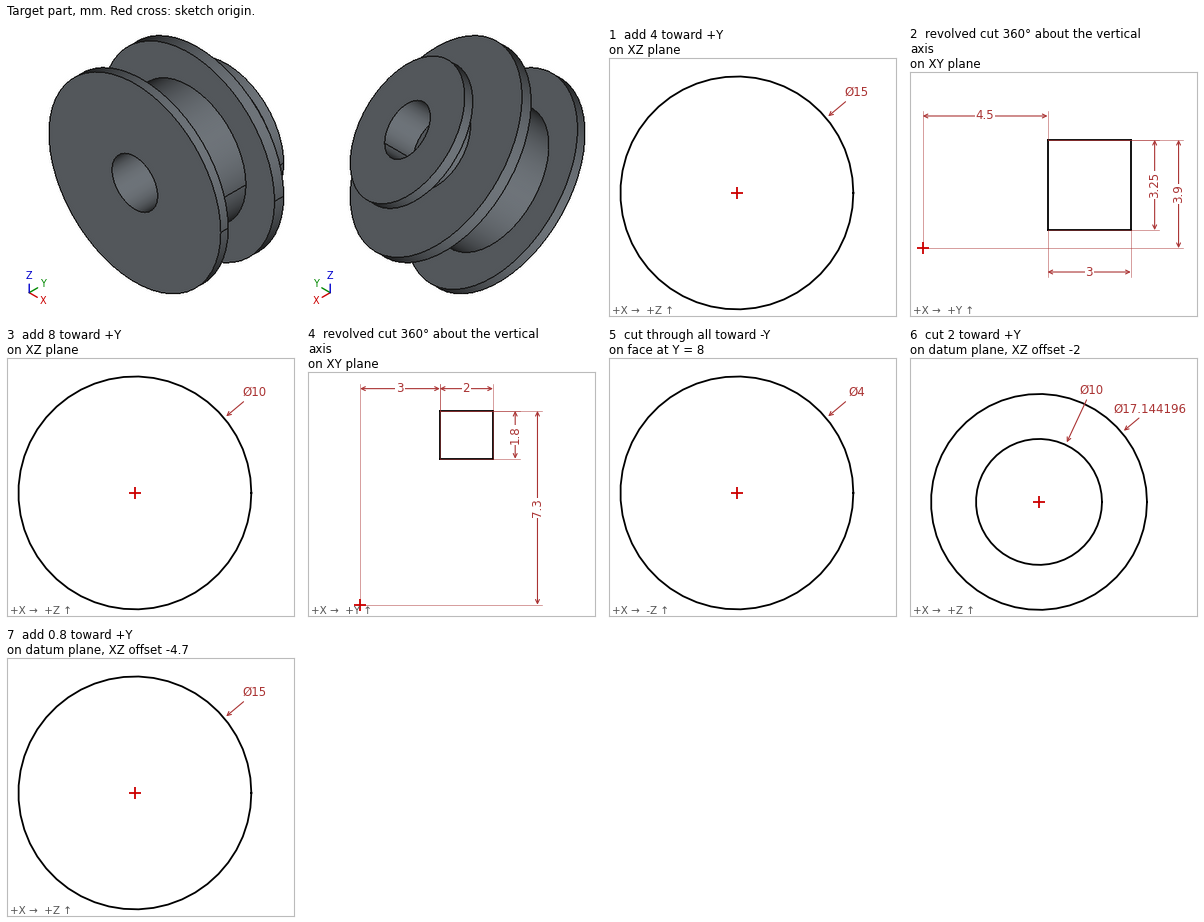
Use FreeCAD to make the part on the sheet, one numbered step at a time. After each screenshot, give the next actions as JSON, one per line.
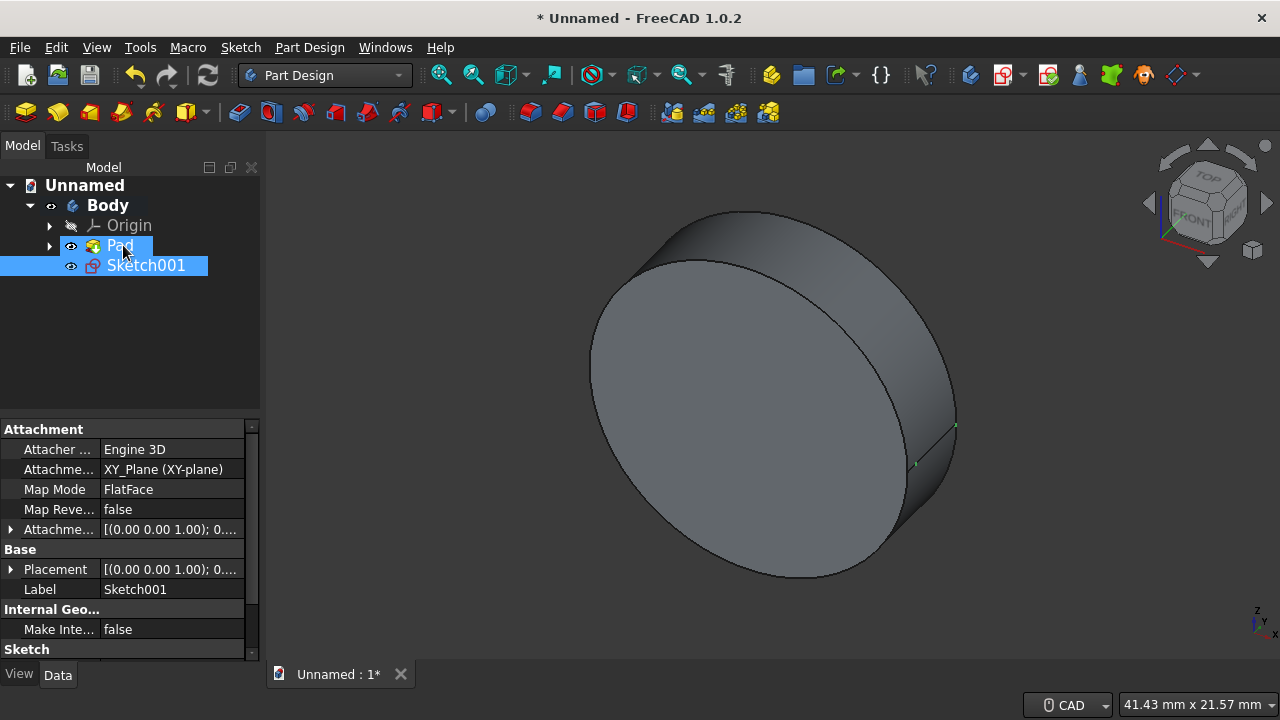
{"action": "left_click", "coordinate": [304, 112]}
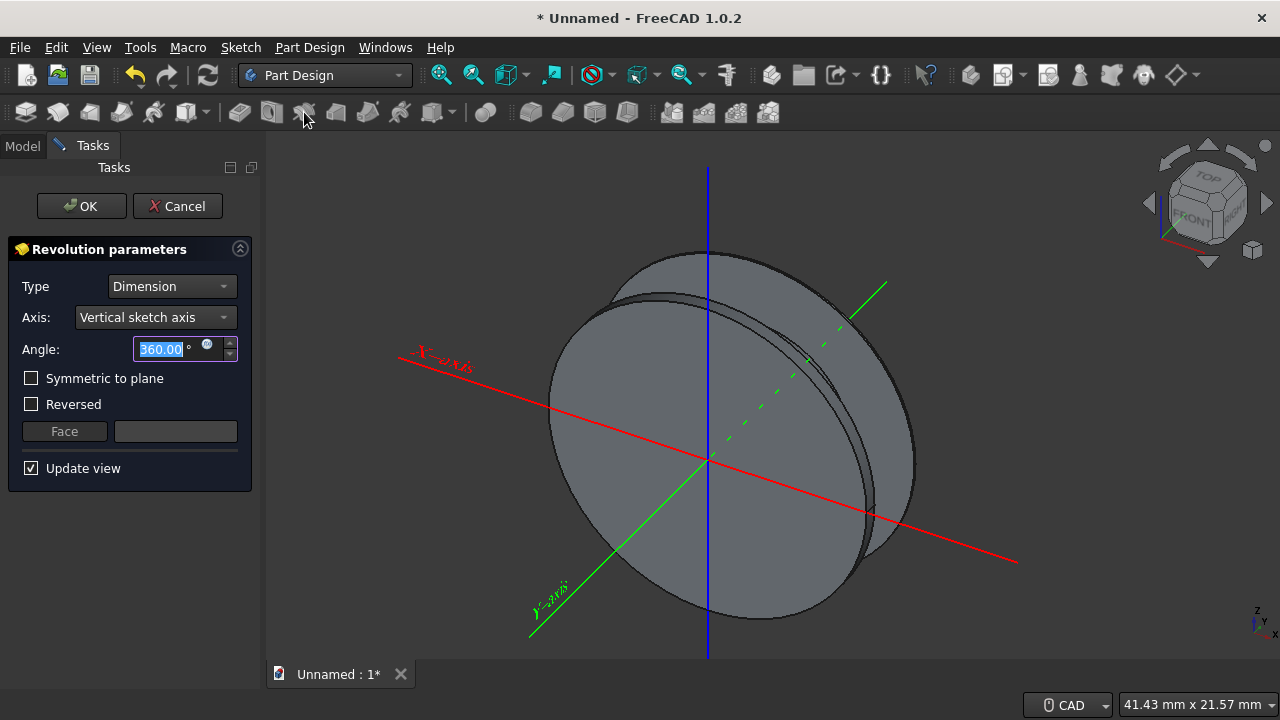
{"action": "left_click", "coordinate": [82, 206]}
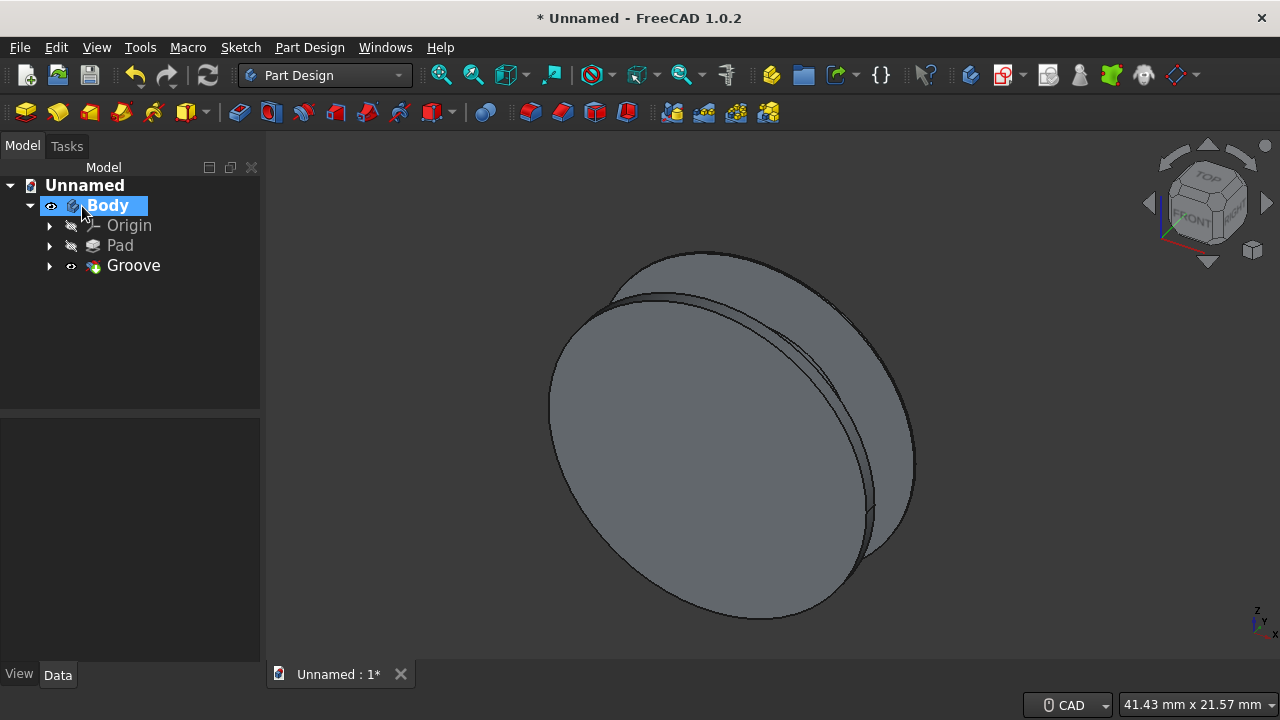
{"action": "left_click", "coordinate": [442, 76]}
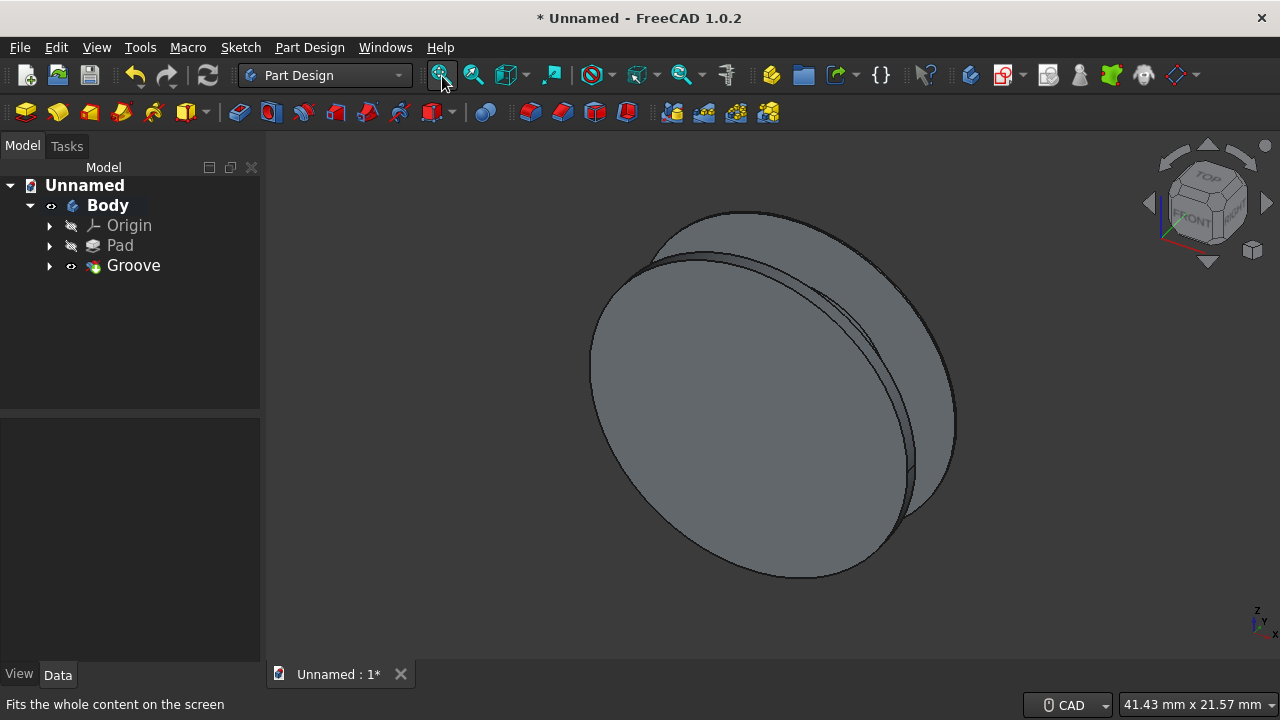
{"action": "left_click", "coordinate": [1004, 76]}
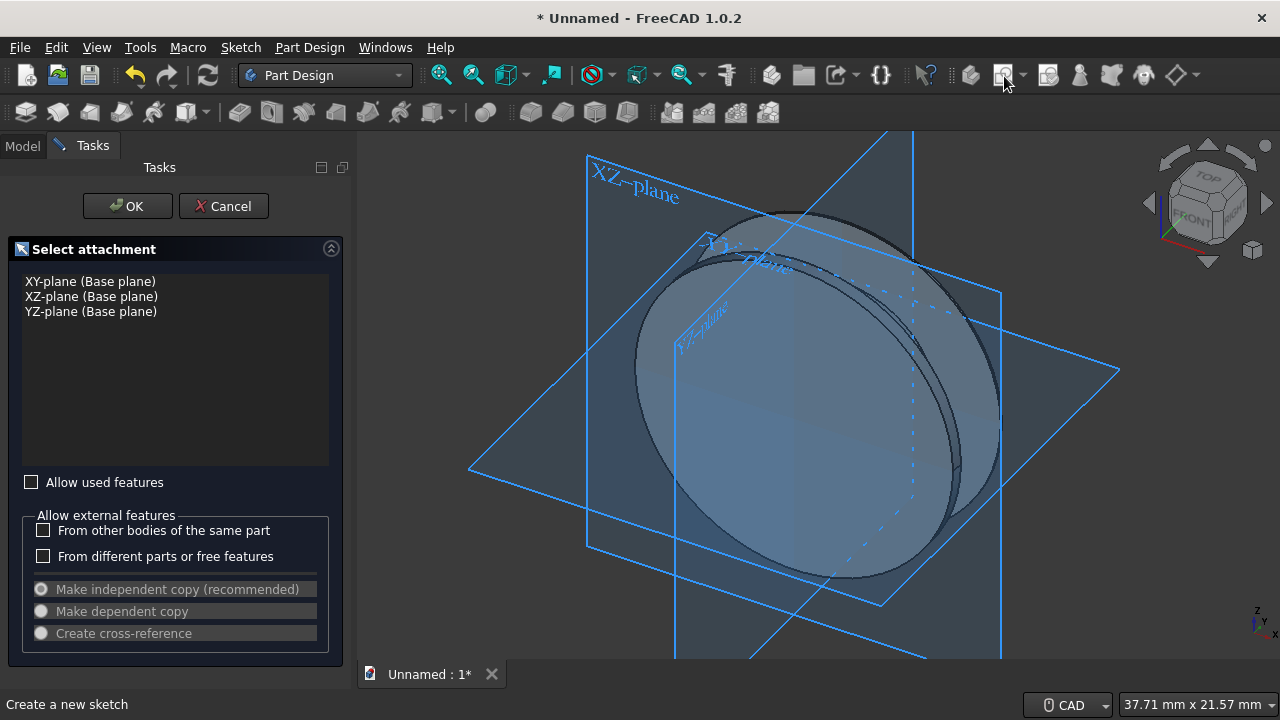
{"action": "left_click", "coordinate": [82, 296]}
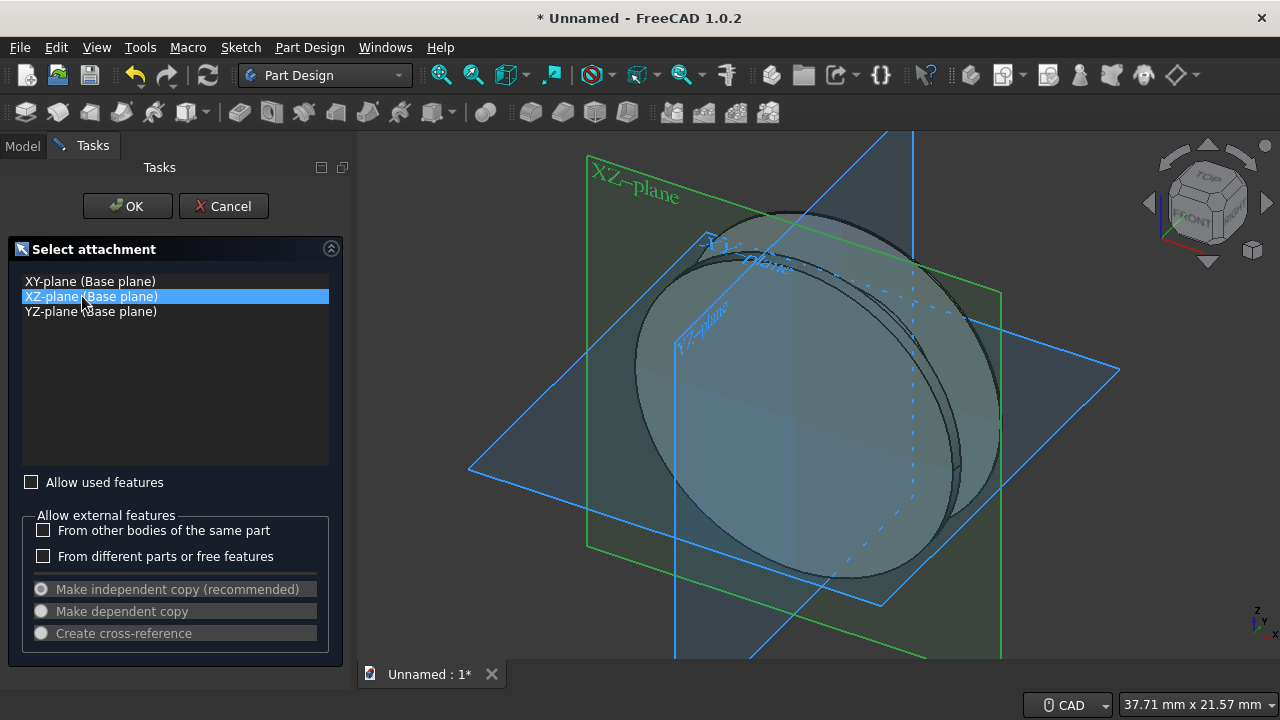
{"action": "left_click", "coordinate": [128, 206]}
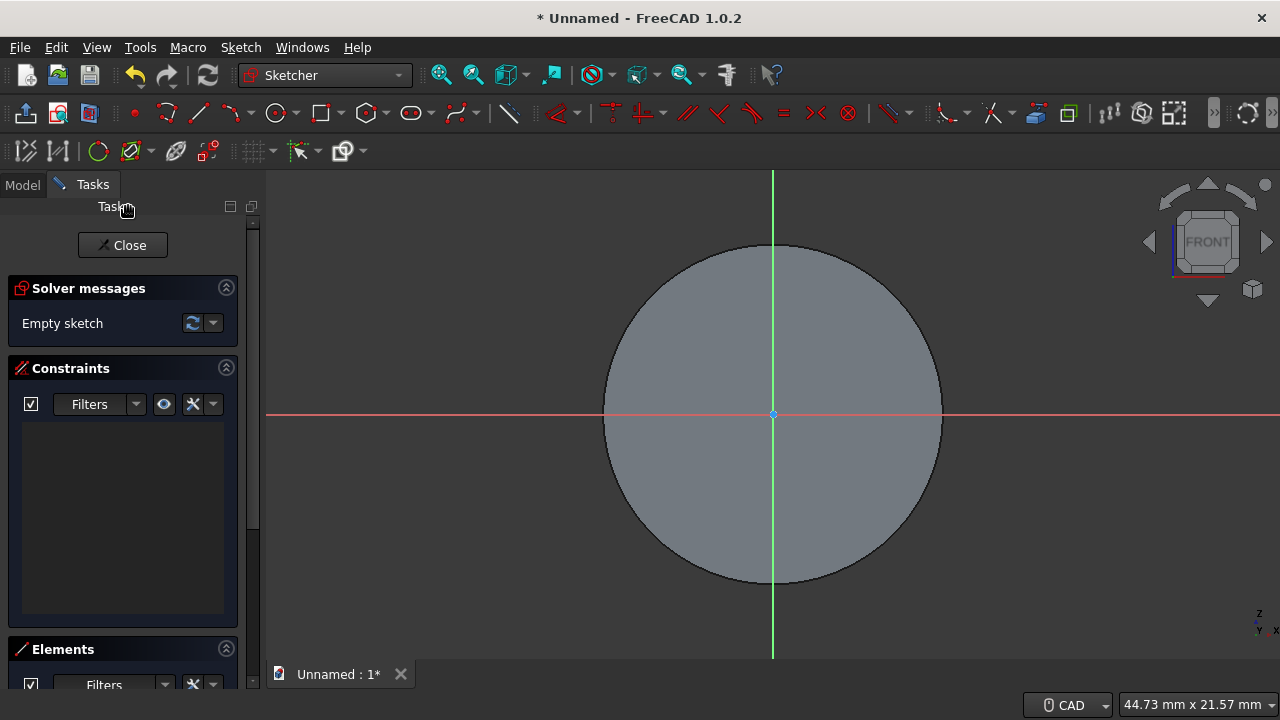
{"action": "left_click", "coordinate": [276, 114]}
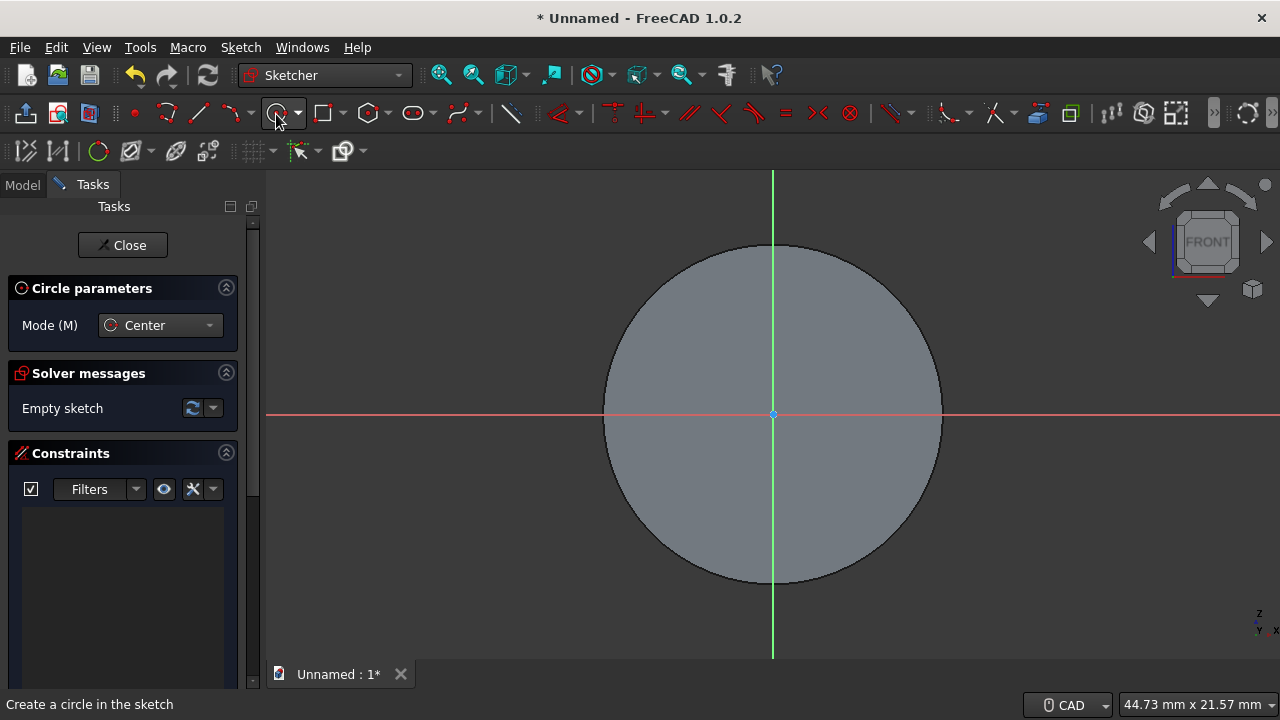
{"action": "left_click", "coordinate": [773, 414]}
{"action": "left_click", "coordinate": [853, 334]}
{"action": "key", "text": "Escape"}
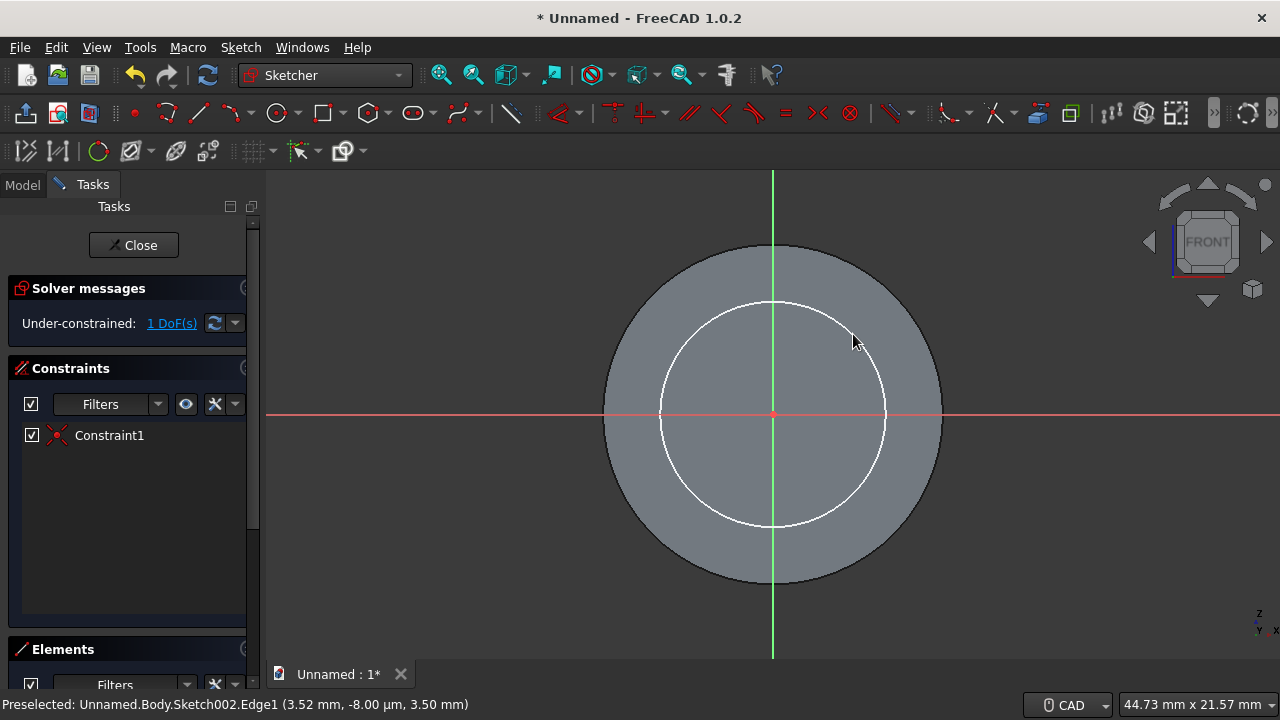
{"action": "left_click", "coordinate": [558, 114]}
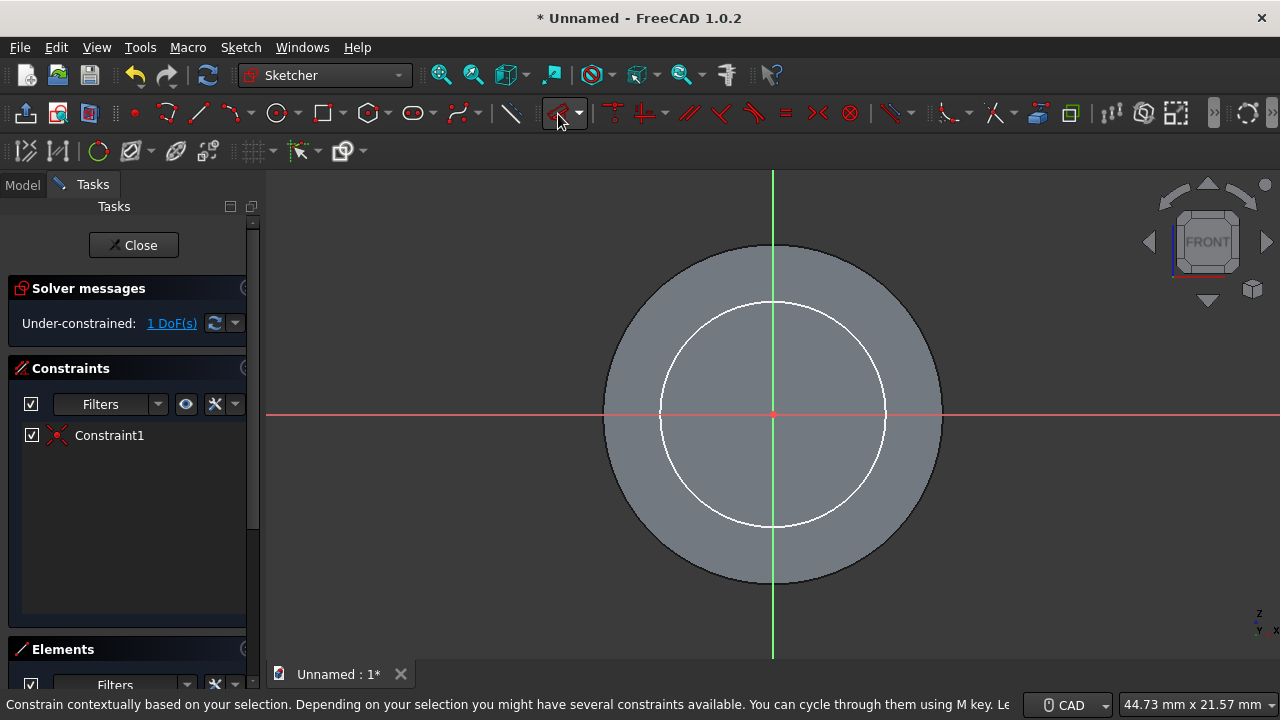
{"action": "left_click", "coordinate": [853, 335]}
{"action": "left_click", "coordinate": [876, 312]}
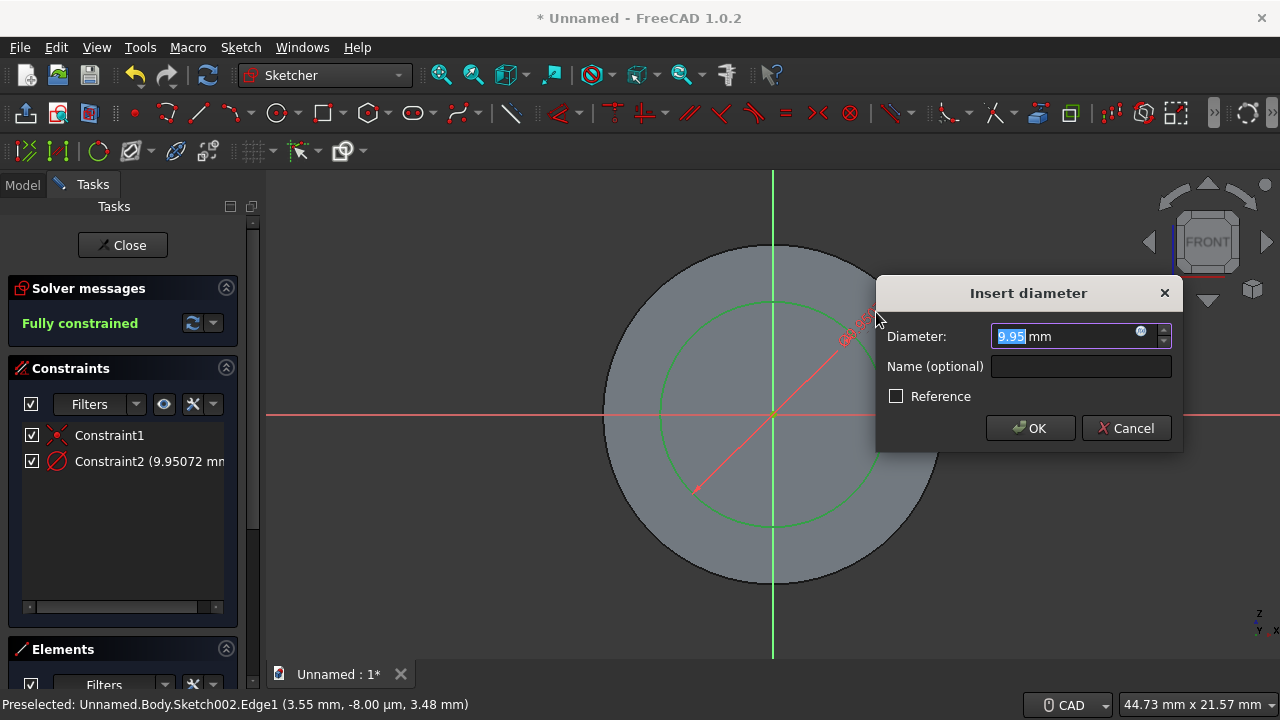
{"action": "type", "text": "10"}
{"action": "key", "text": "Return"}
{"action": "key", "text": "Escape"}